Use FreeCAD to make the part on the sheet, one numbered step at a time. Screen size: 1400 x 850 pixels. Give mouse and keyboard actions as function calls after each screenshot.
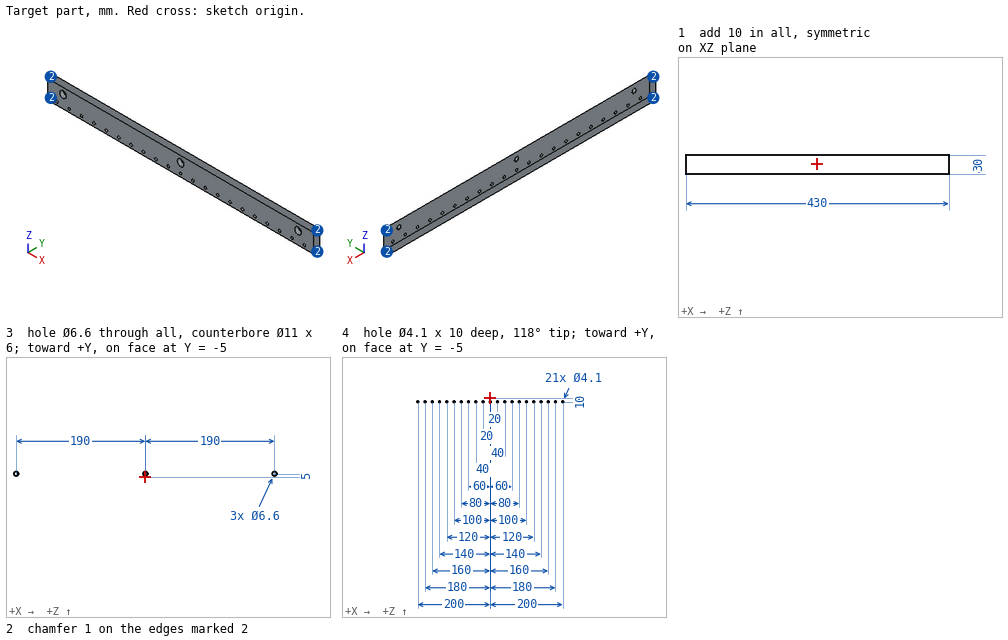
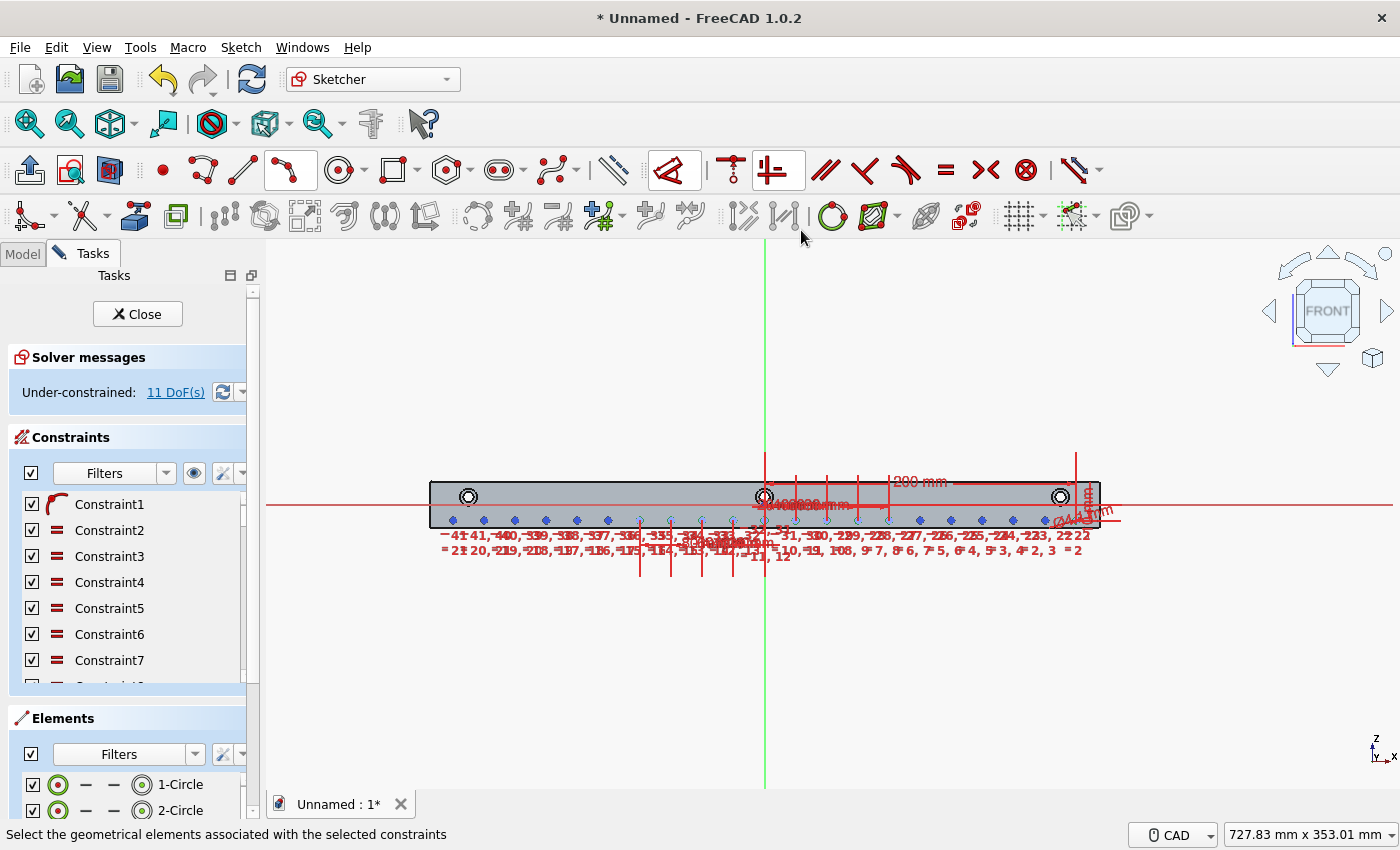
click(1045, 521)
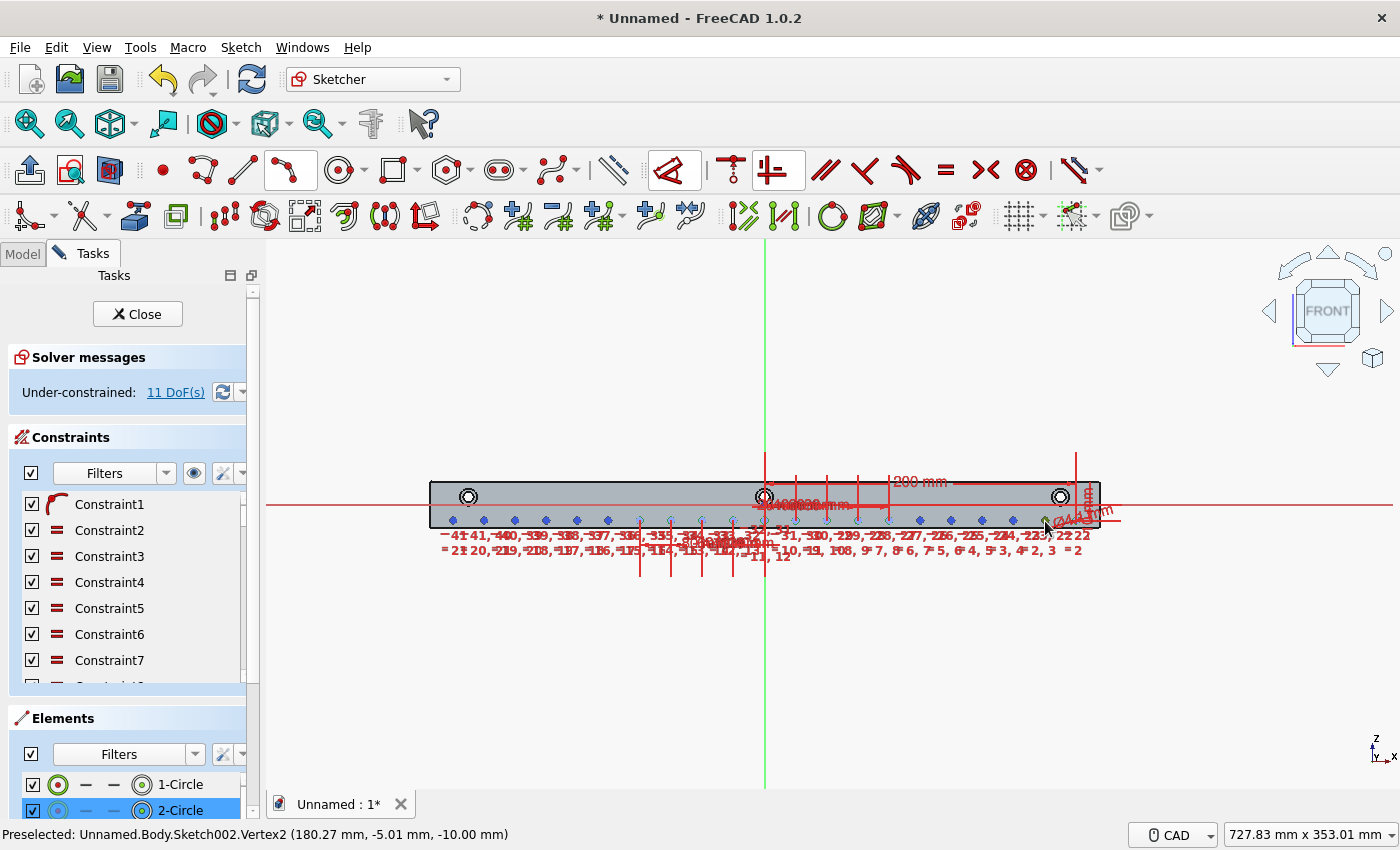
key(l)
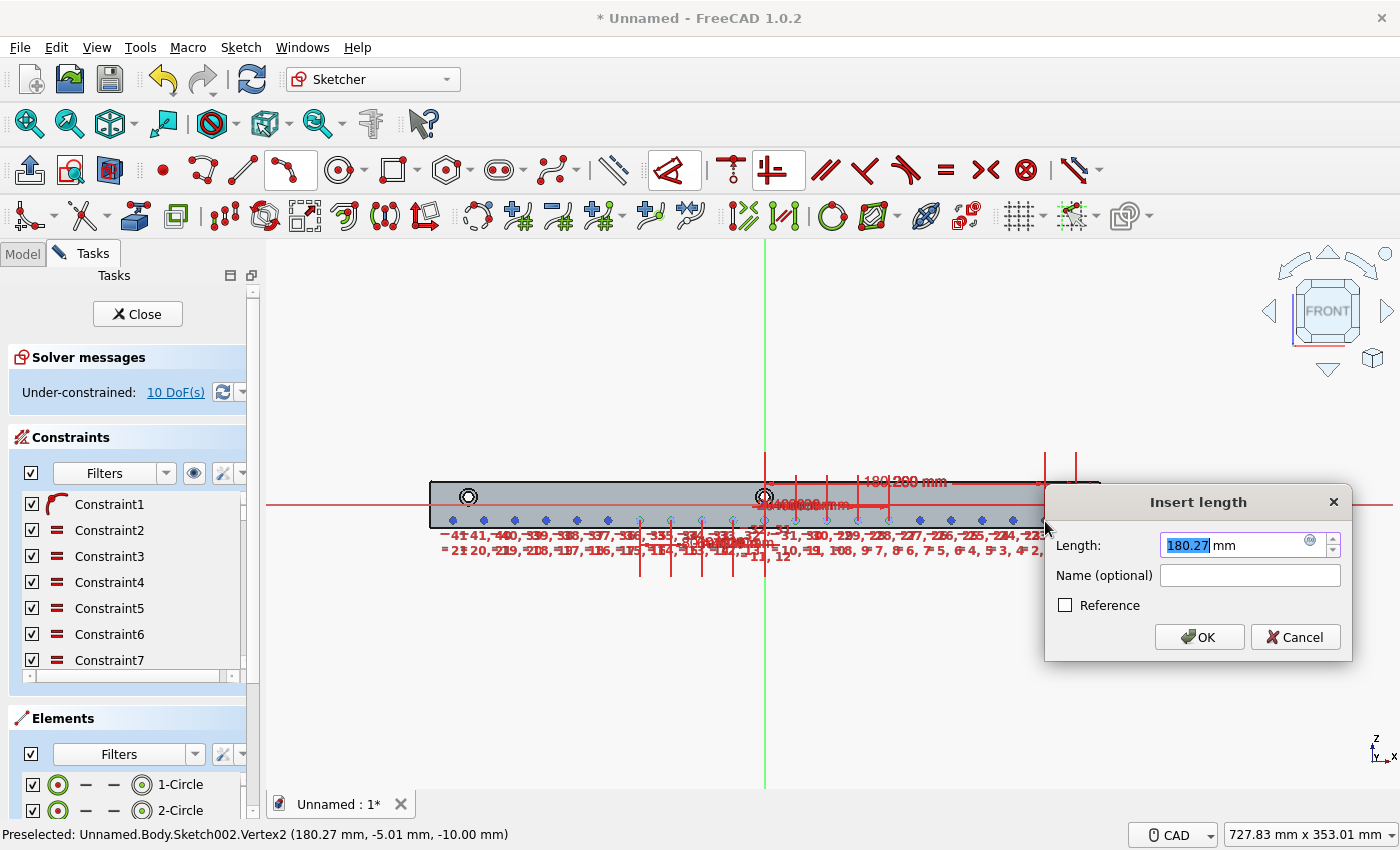
text(180)
key(Return)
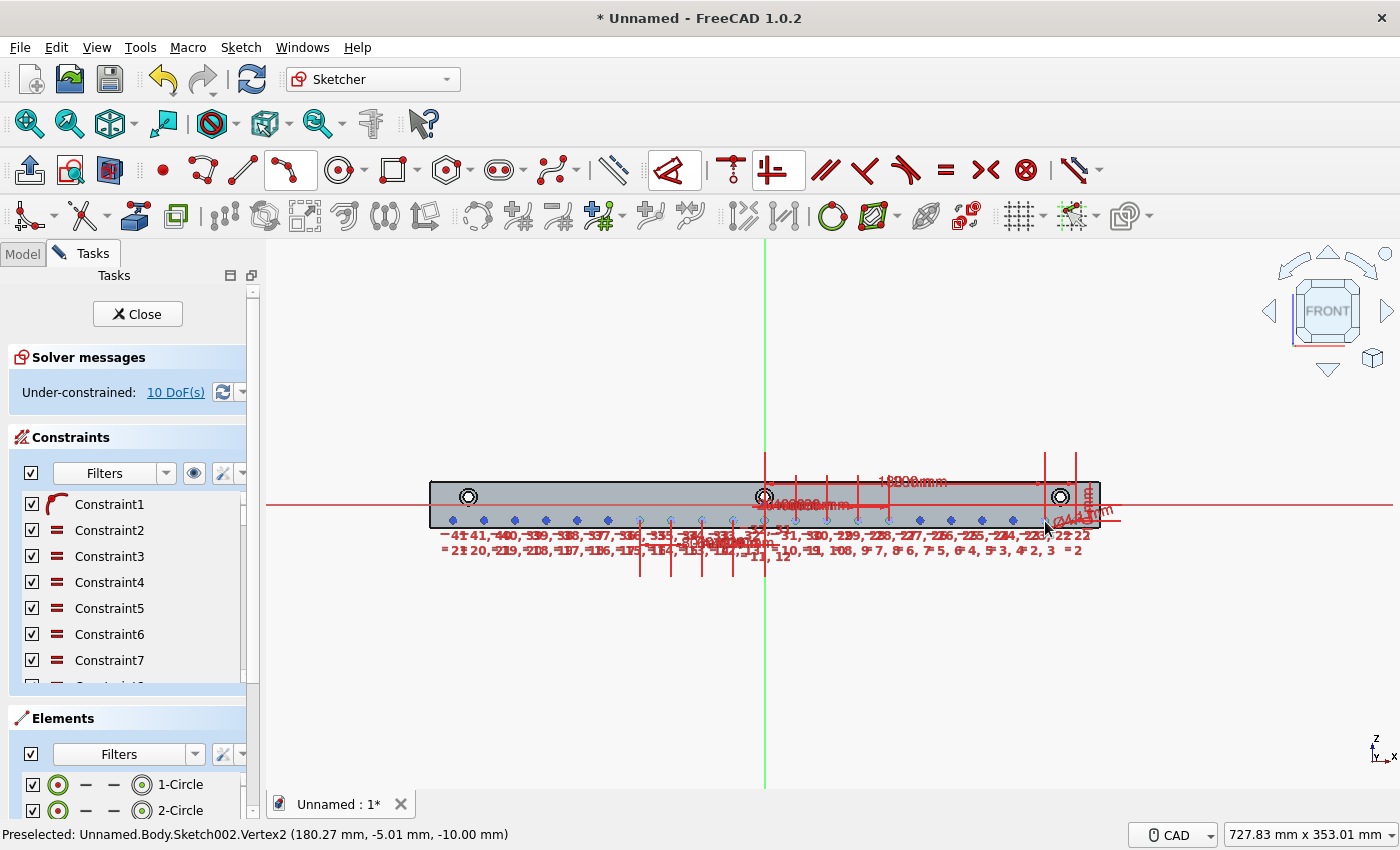
click(1013, 521)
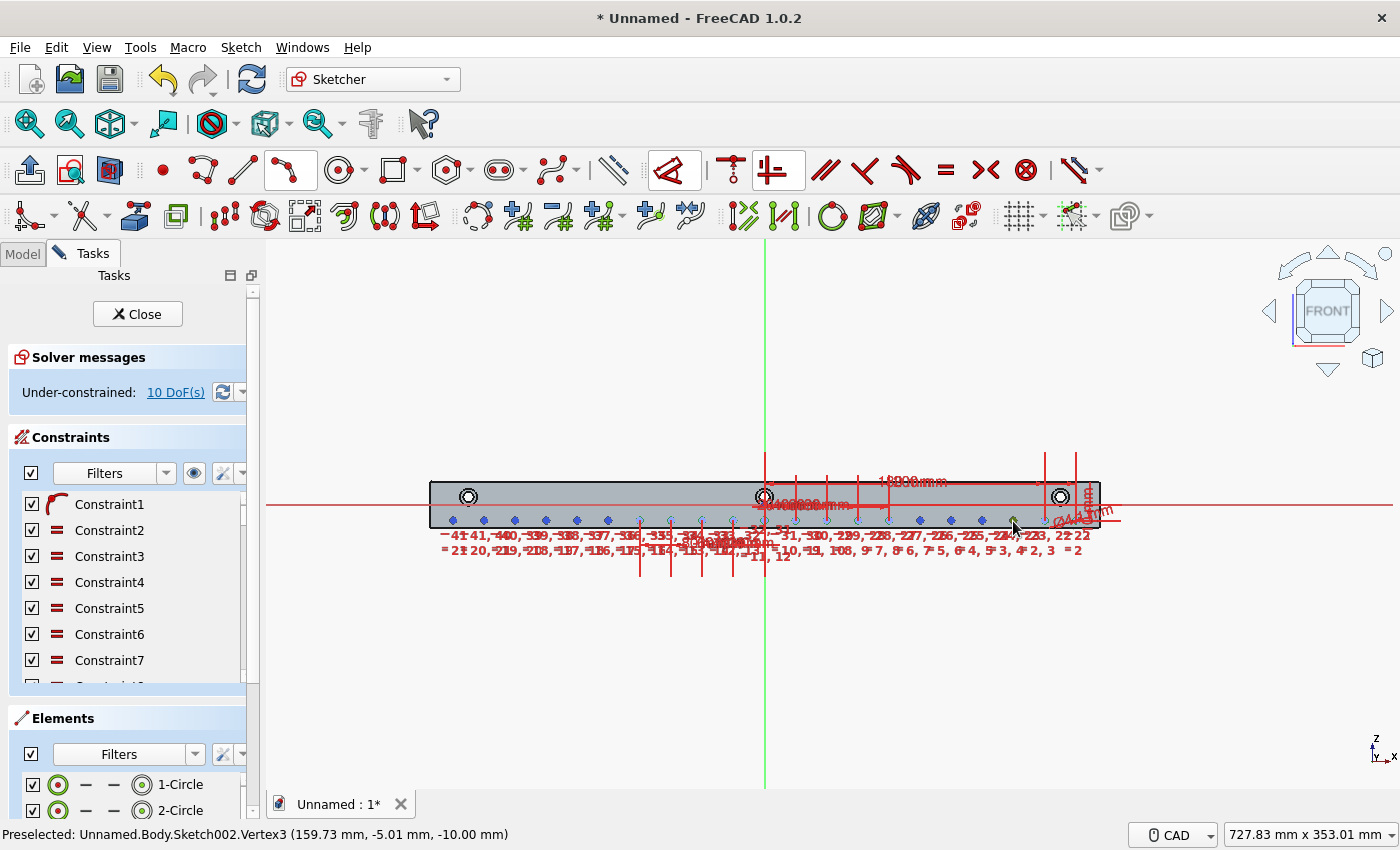
key(l)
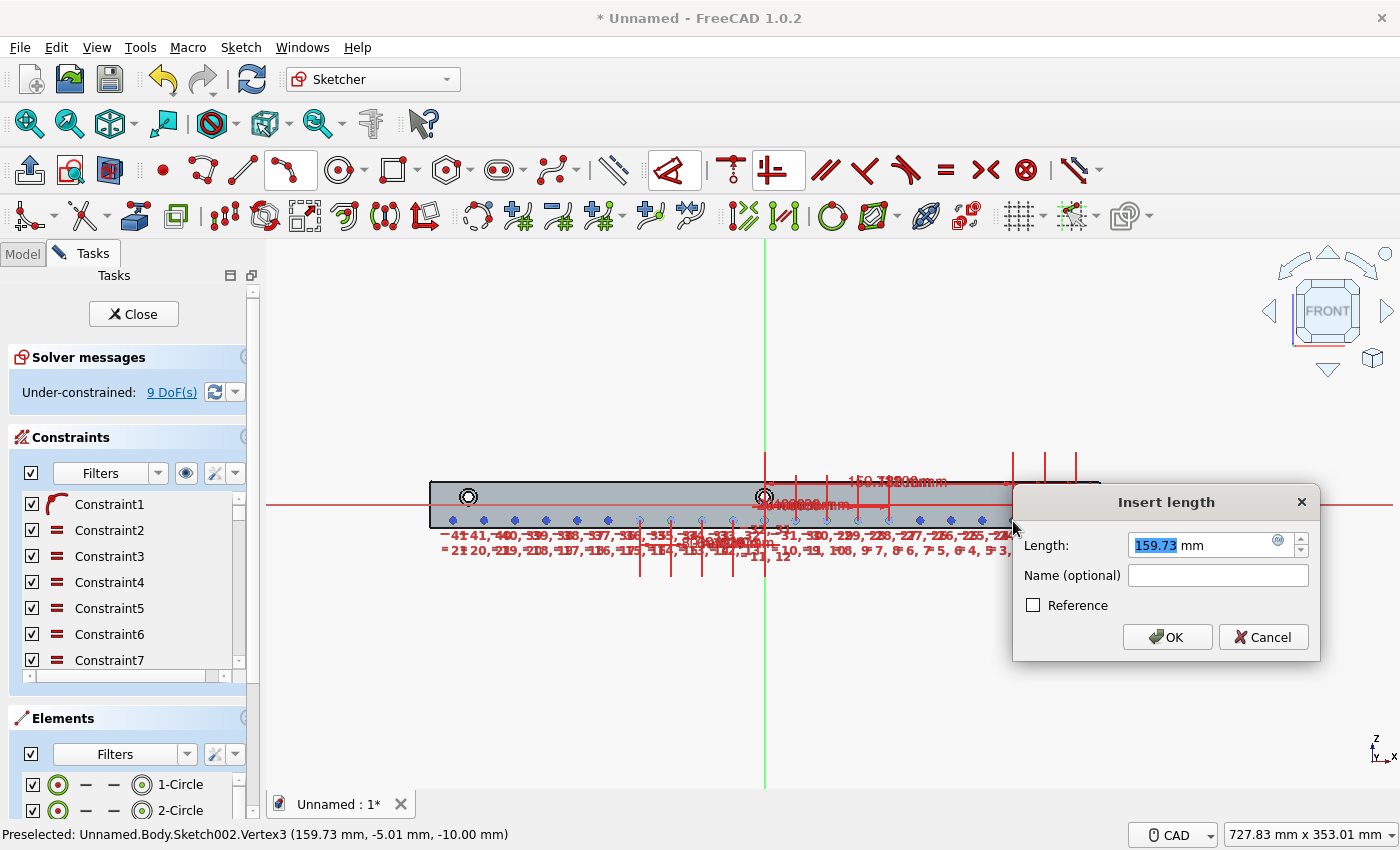
text(160)
key(Return)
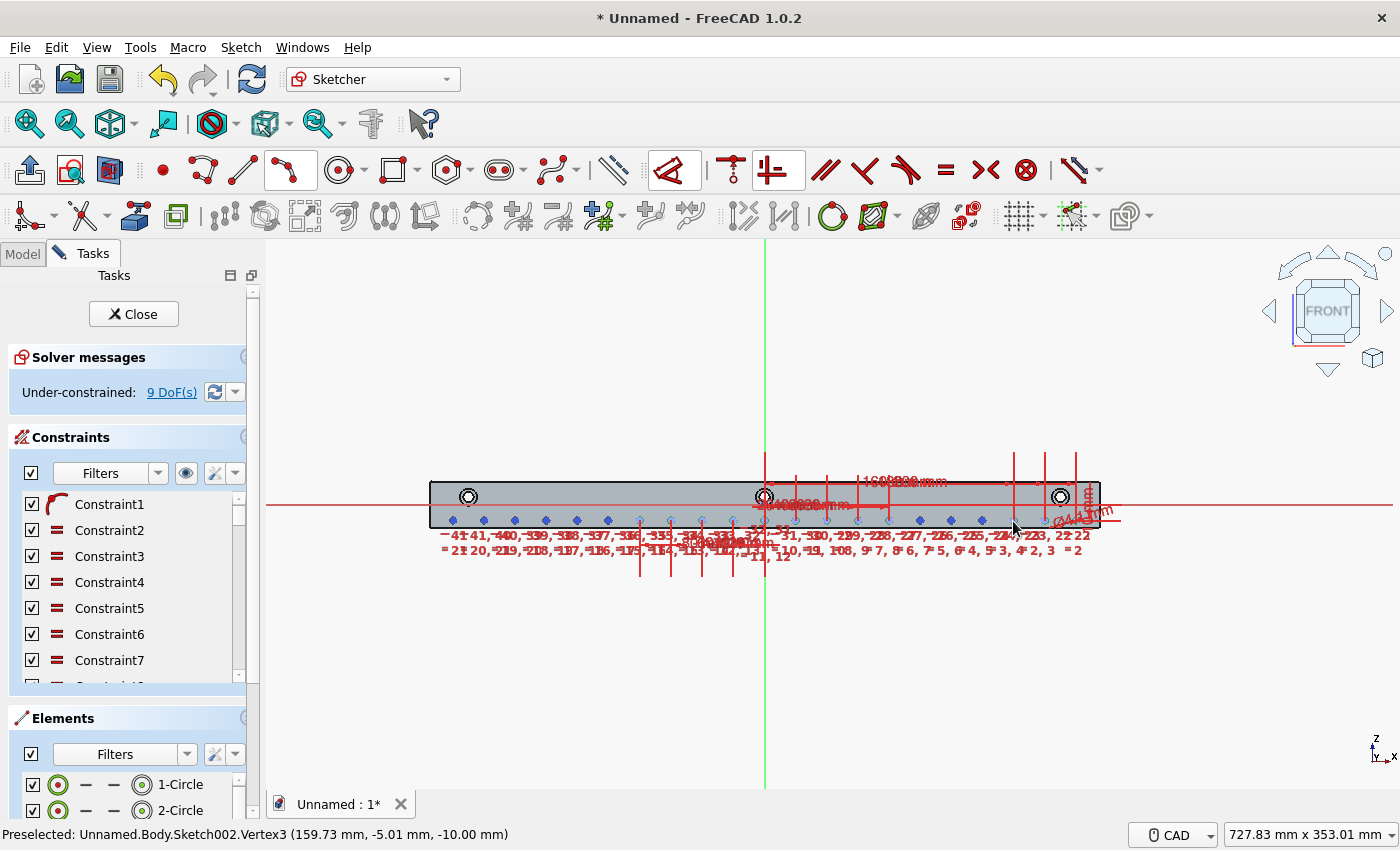
click(982, 521)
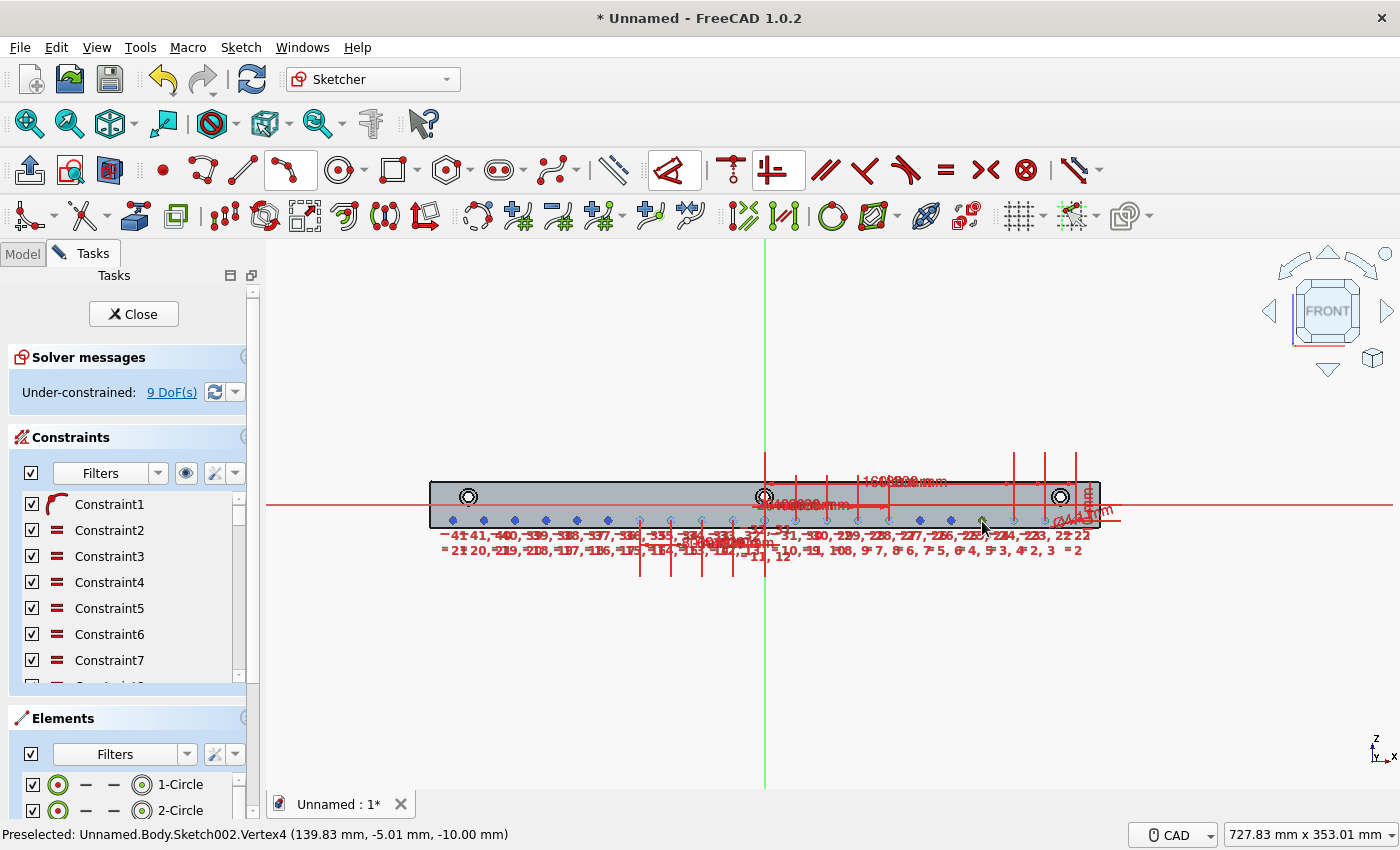
click(696, 170)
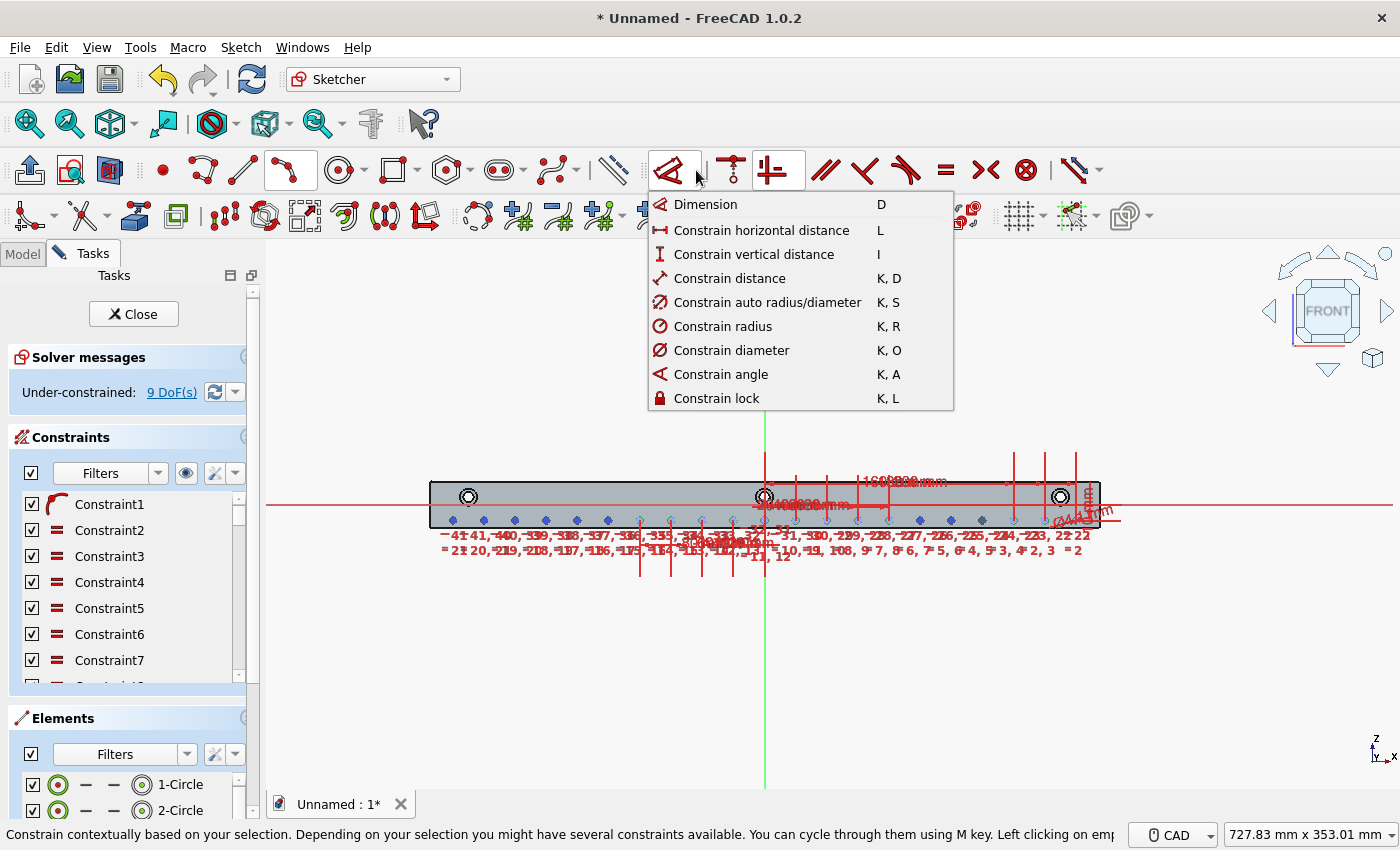
click(801, 230)